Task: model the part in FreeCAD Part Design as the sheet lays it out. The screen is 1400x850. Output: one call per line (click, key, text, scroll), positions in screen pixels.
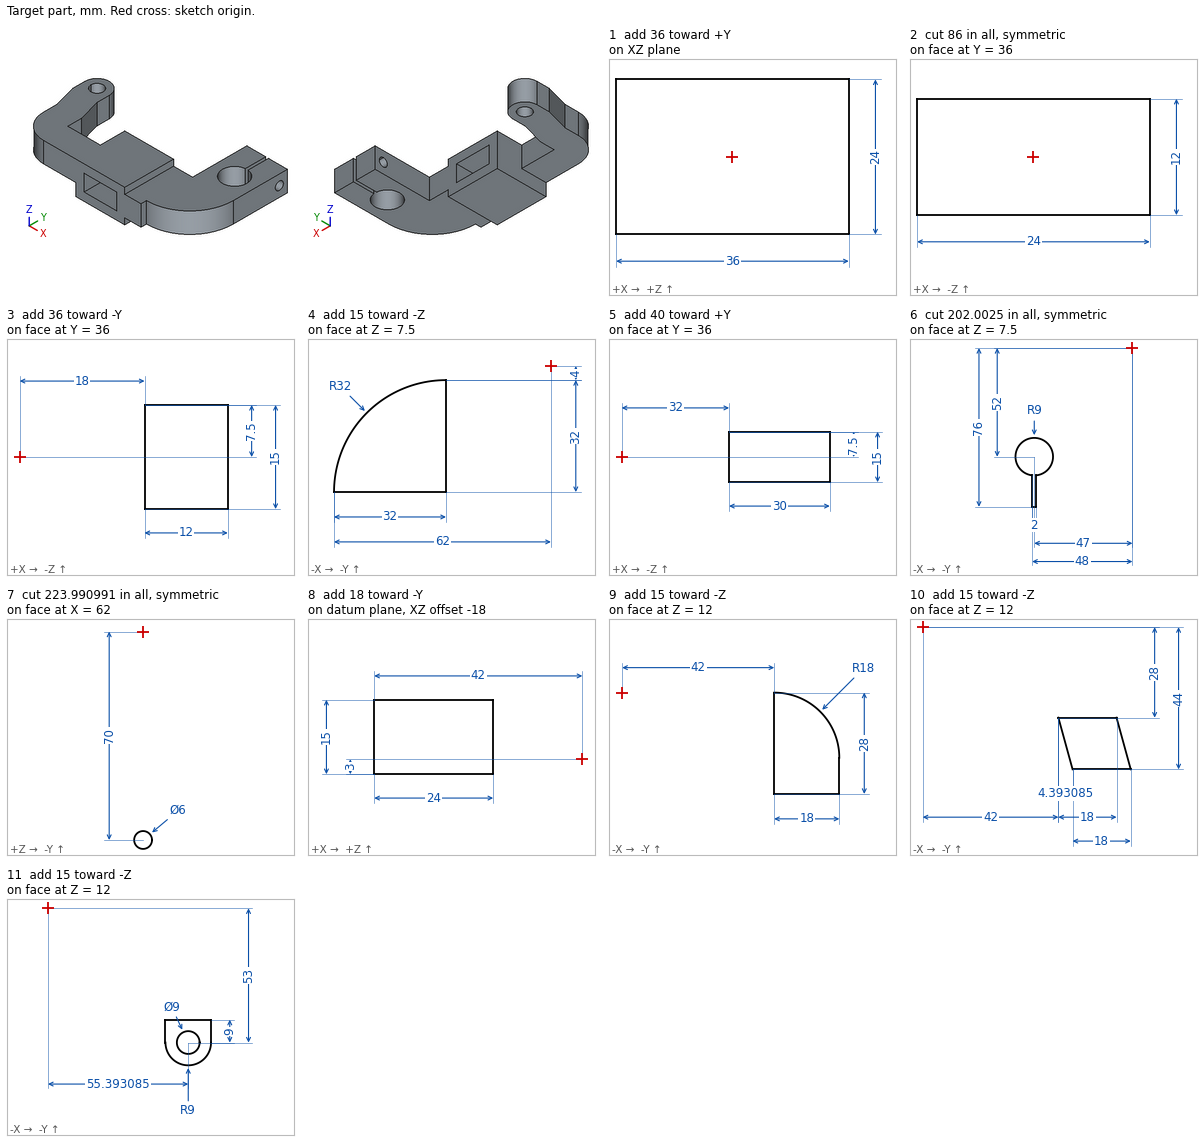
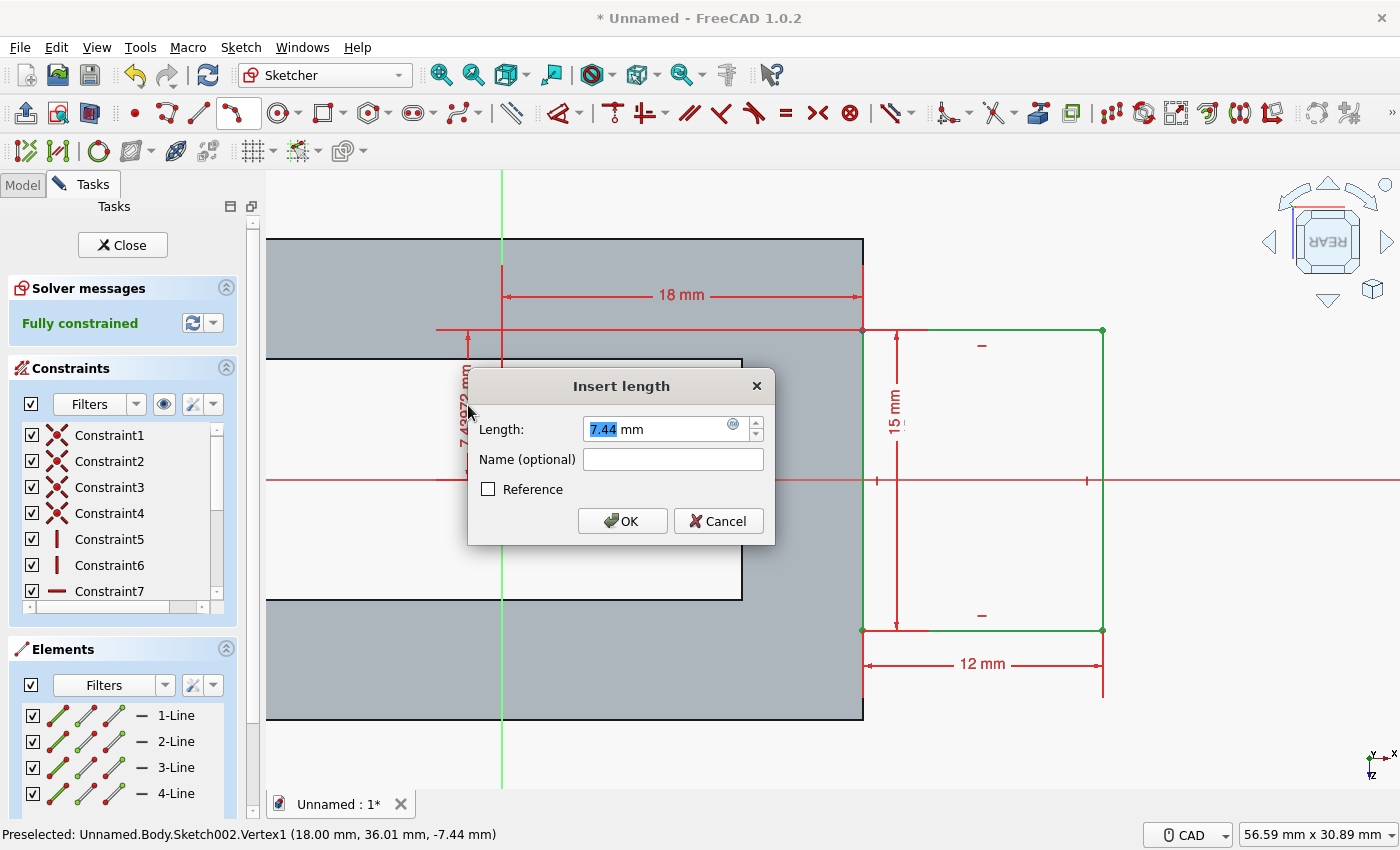
text(7.5)
key(Return)
key(Escape)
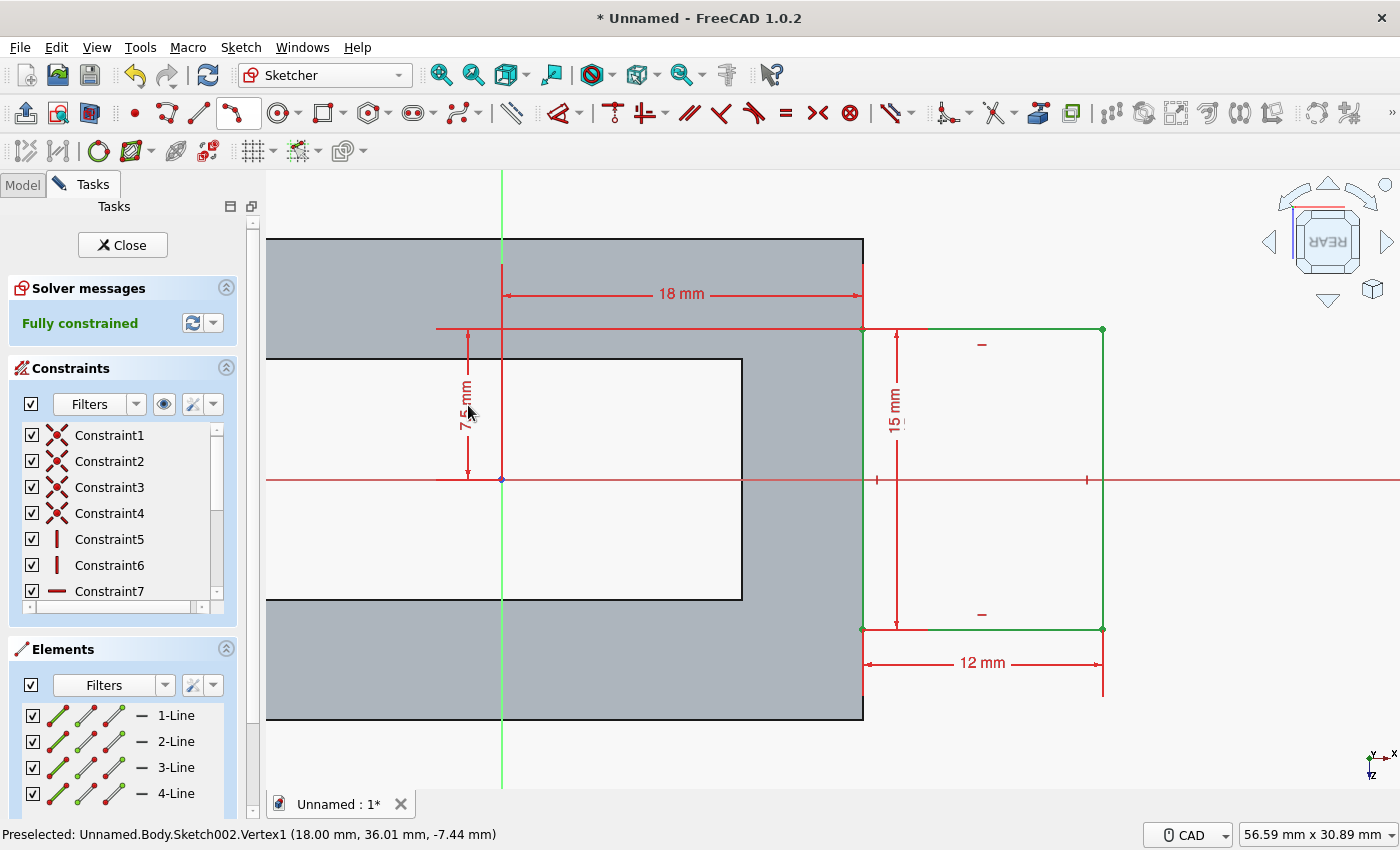
click(123, 245)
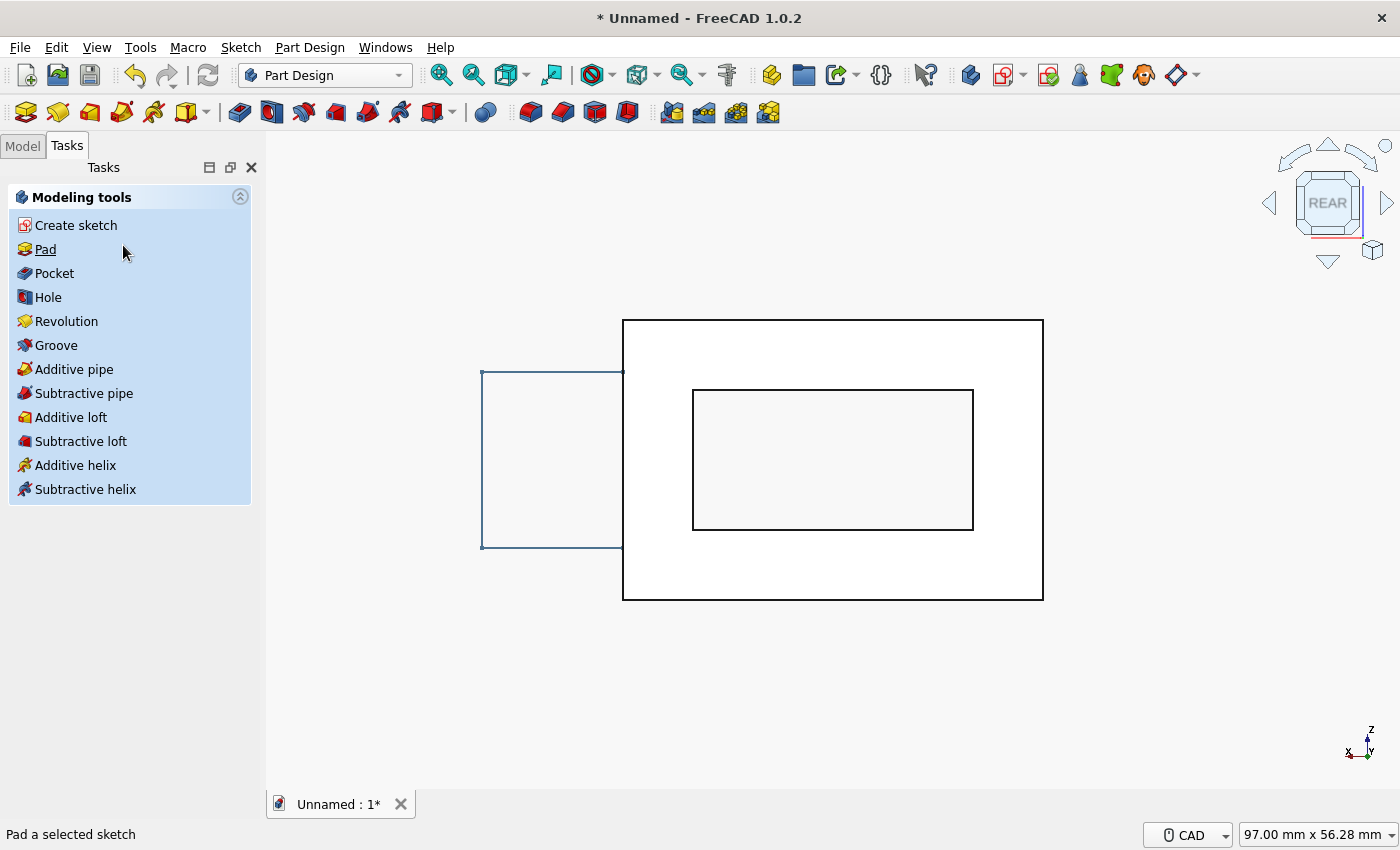
click(26, 112)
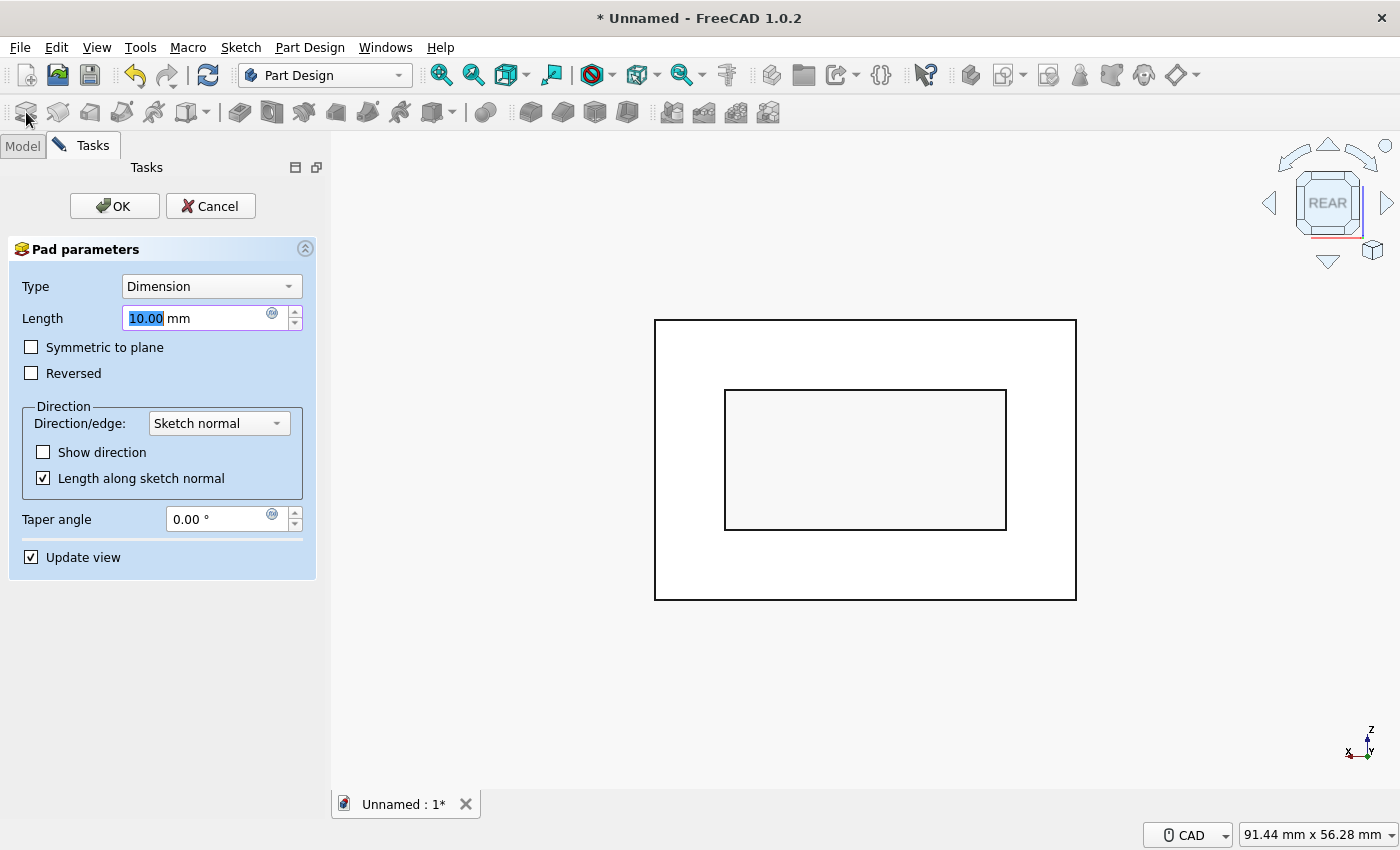
text(36)
key(Tab)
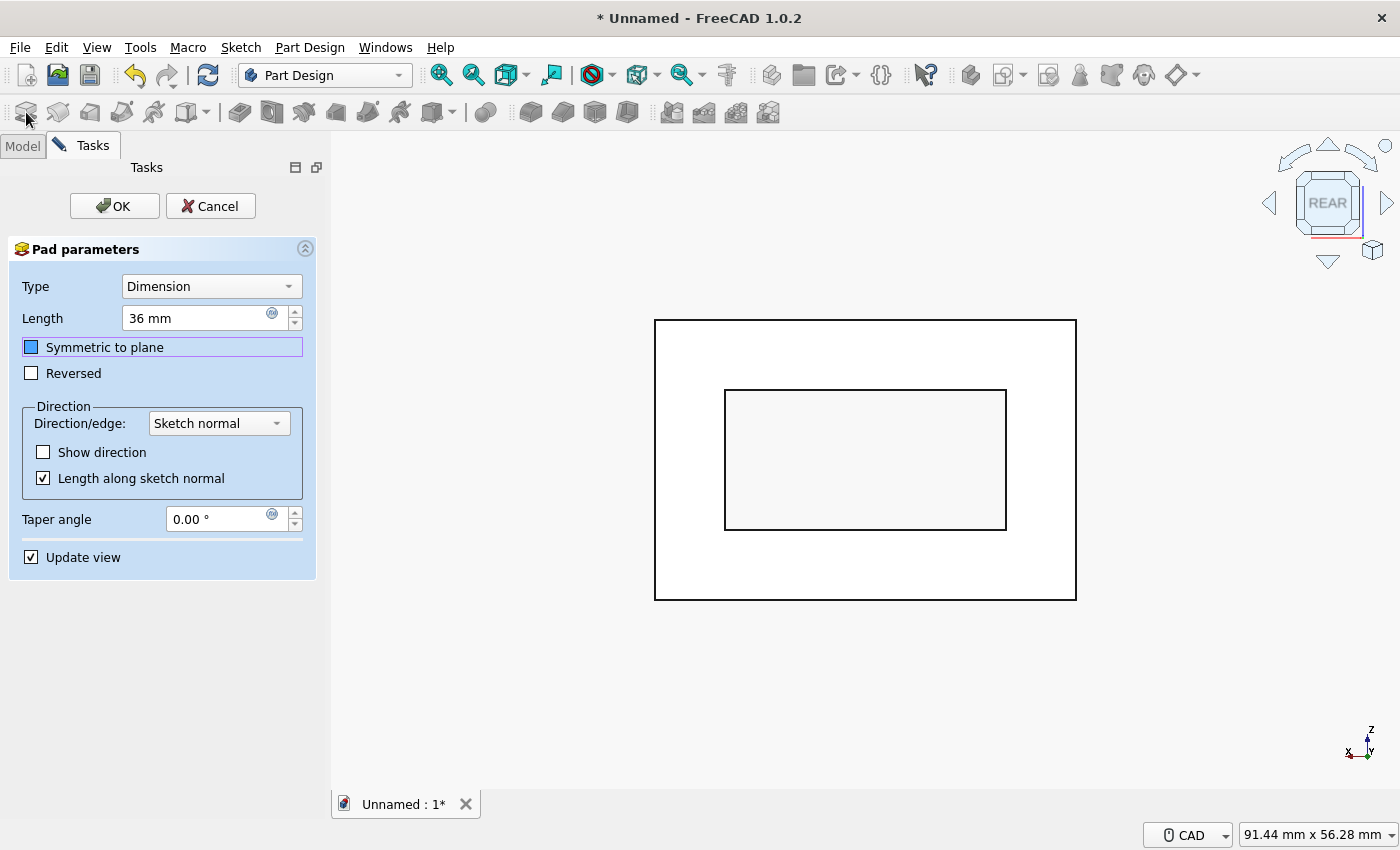
click(30, 373)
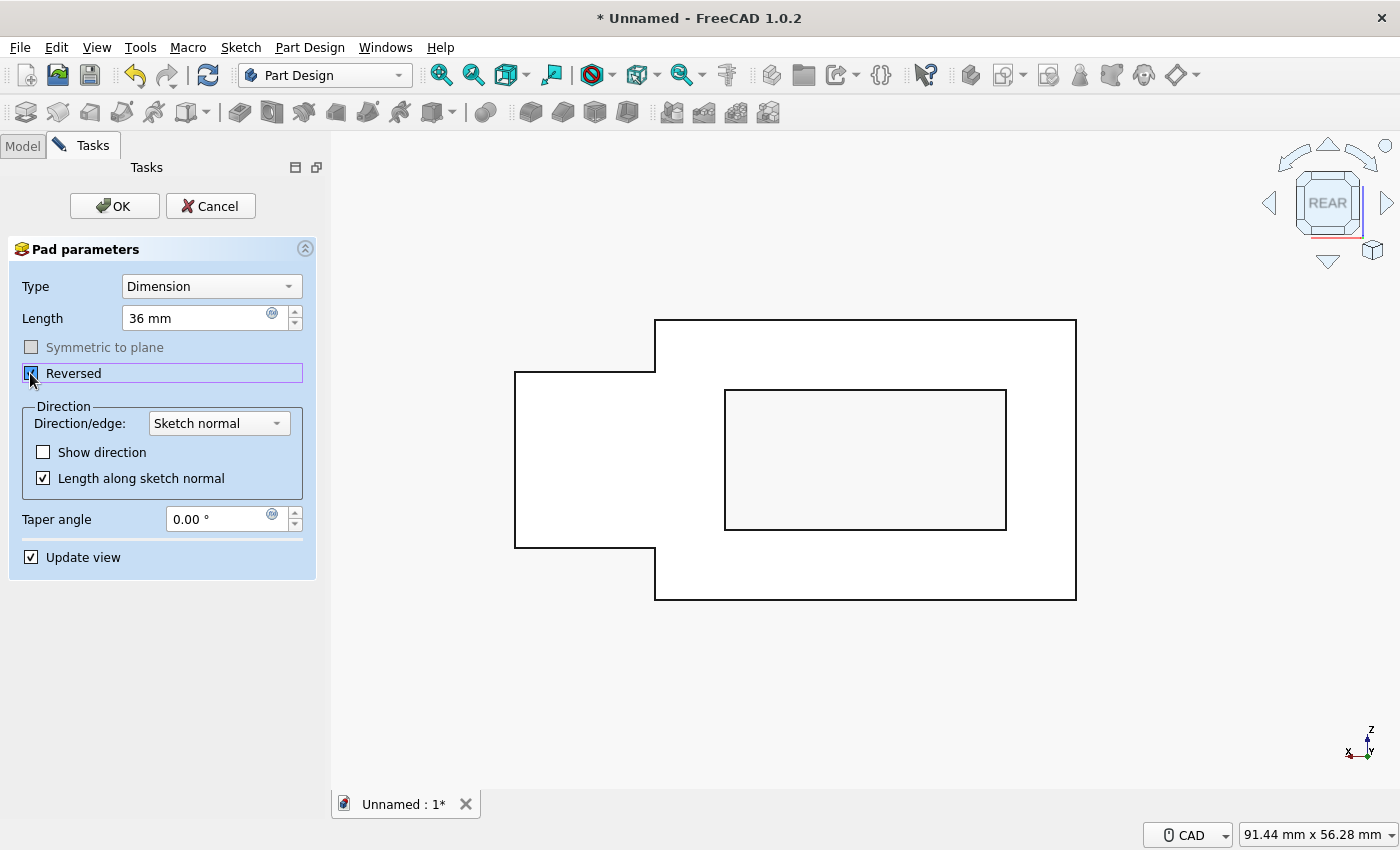
click(115, 206)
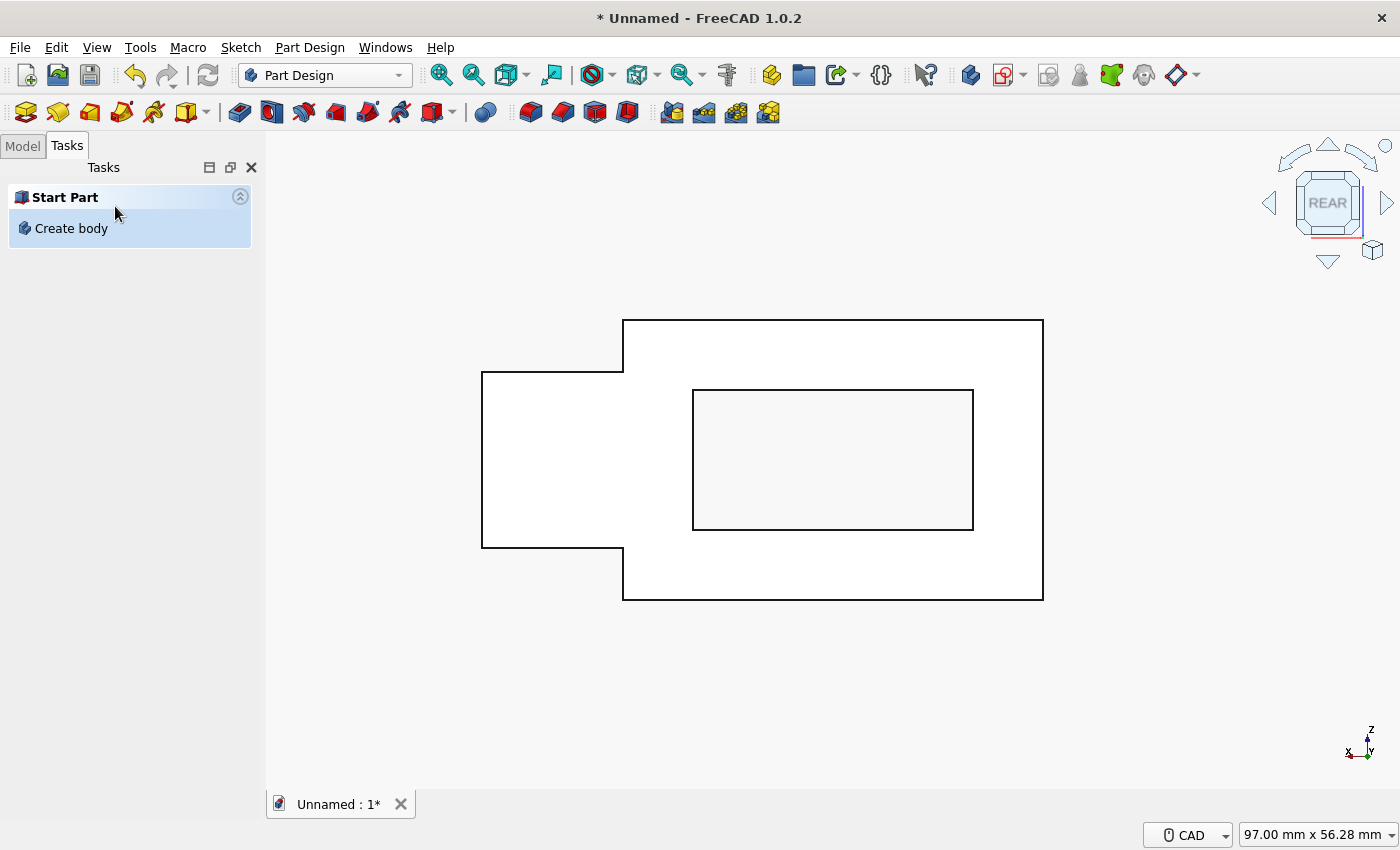
key(0)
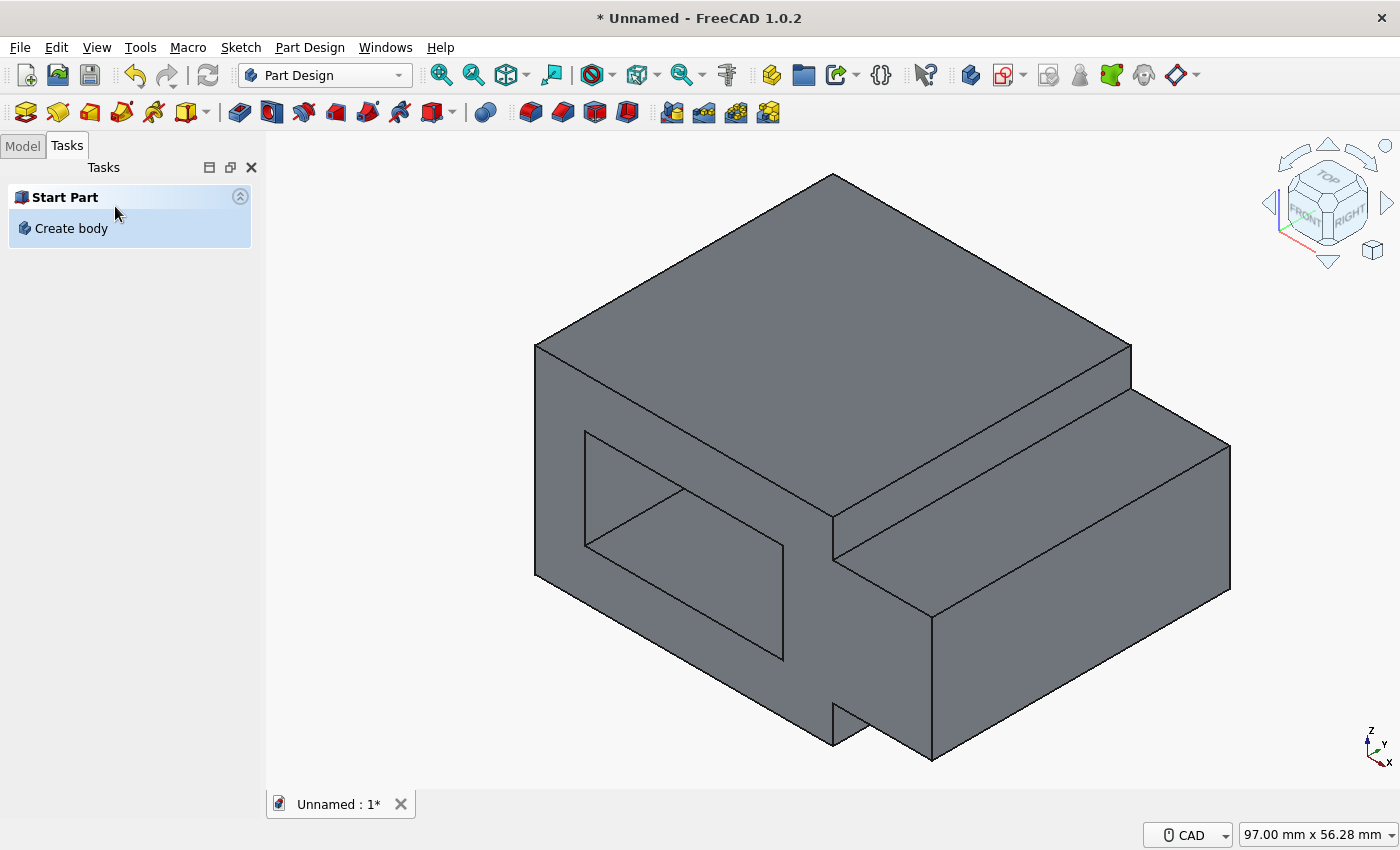
key(v)
key(f)